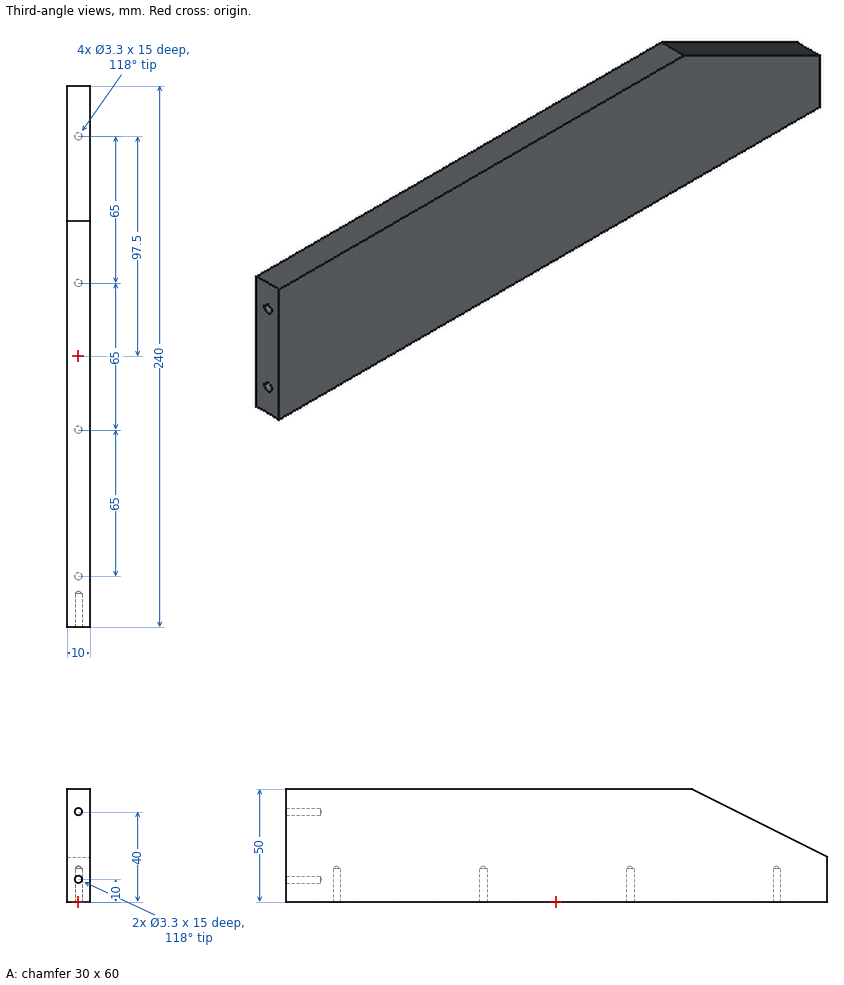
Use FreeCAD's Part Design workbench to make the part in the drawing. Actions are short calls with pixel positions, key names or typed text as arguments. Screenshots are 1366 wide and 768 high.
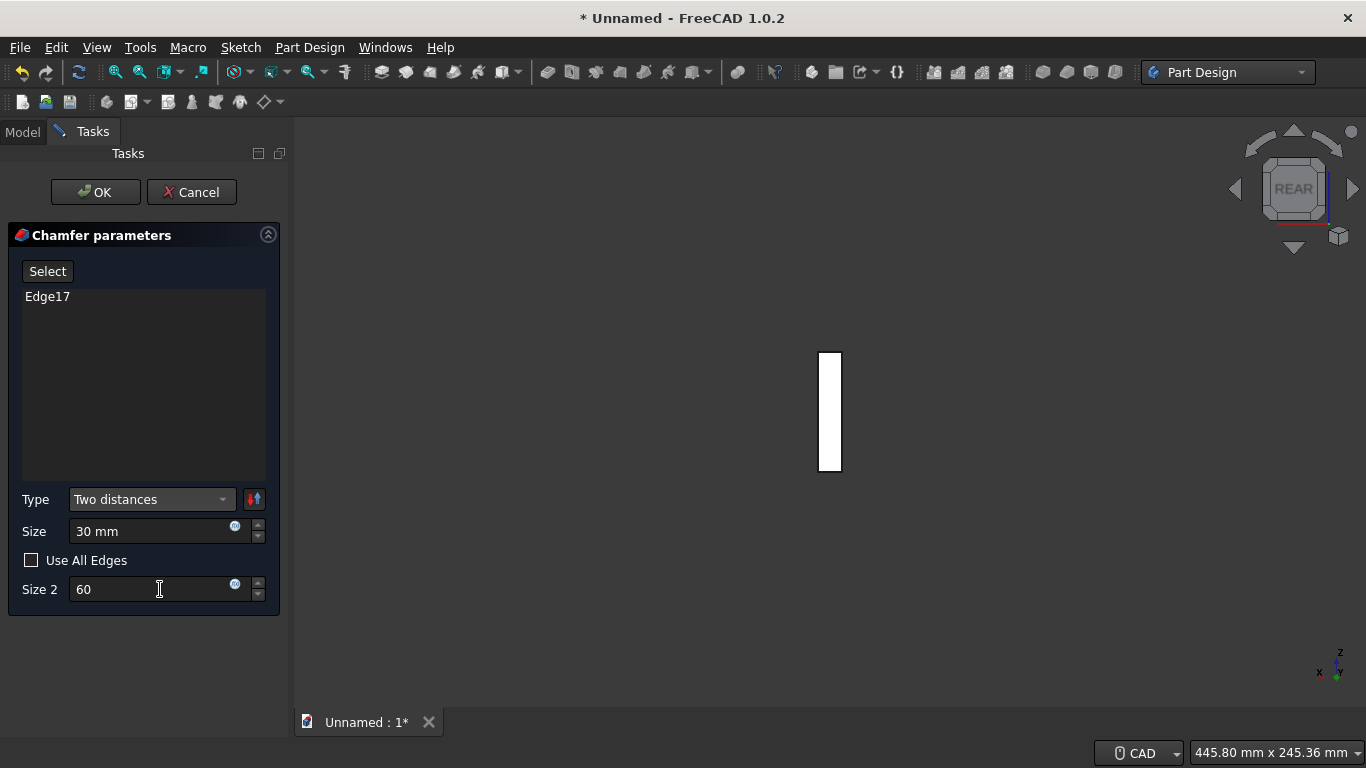
click(254, 500)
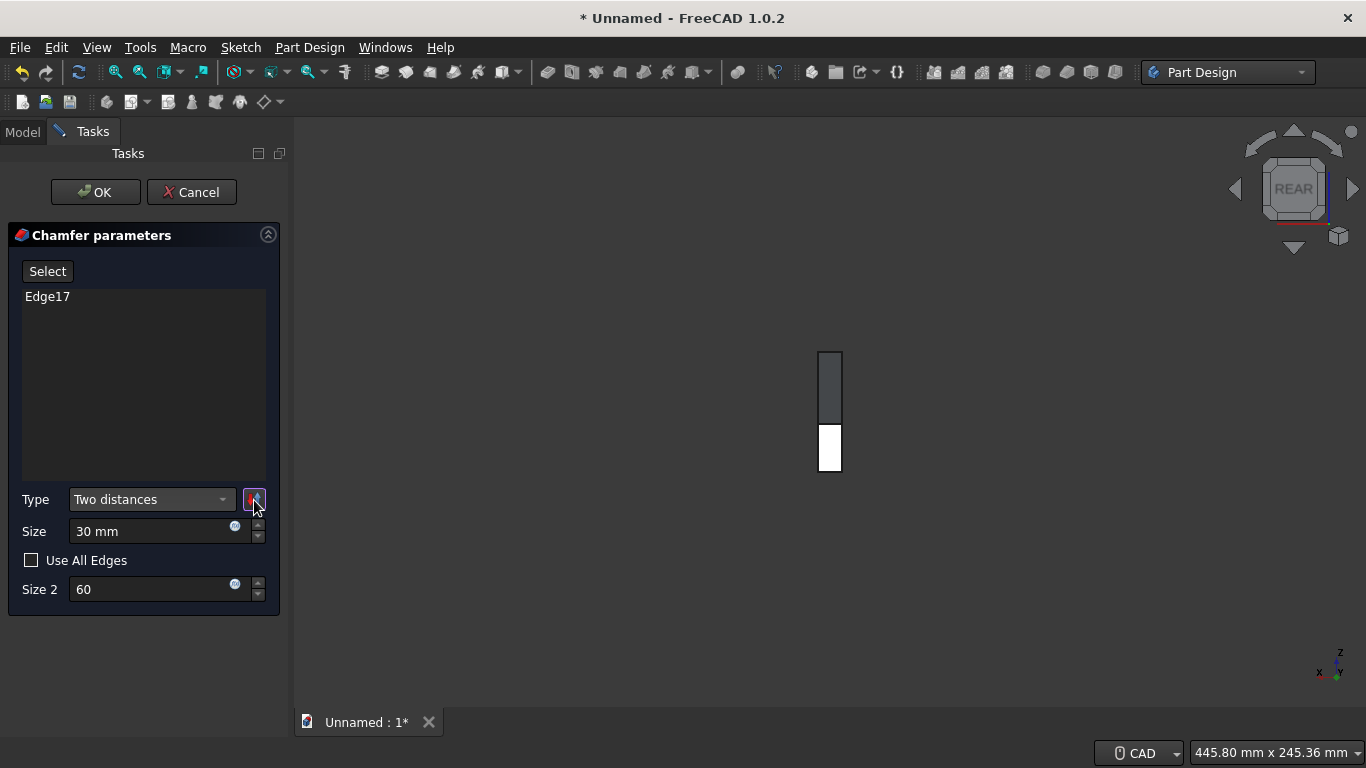
click(96, 192)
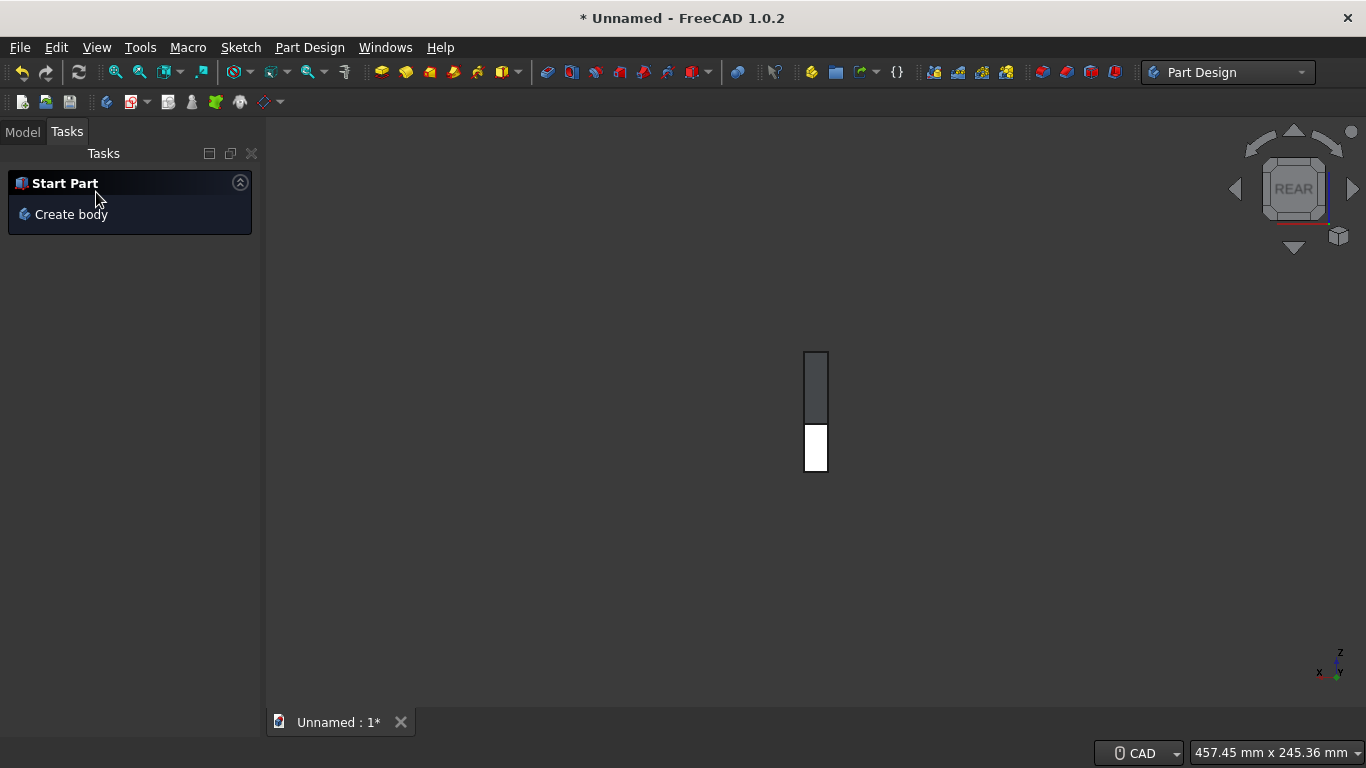
key(0)